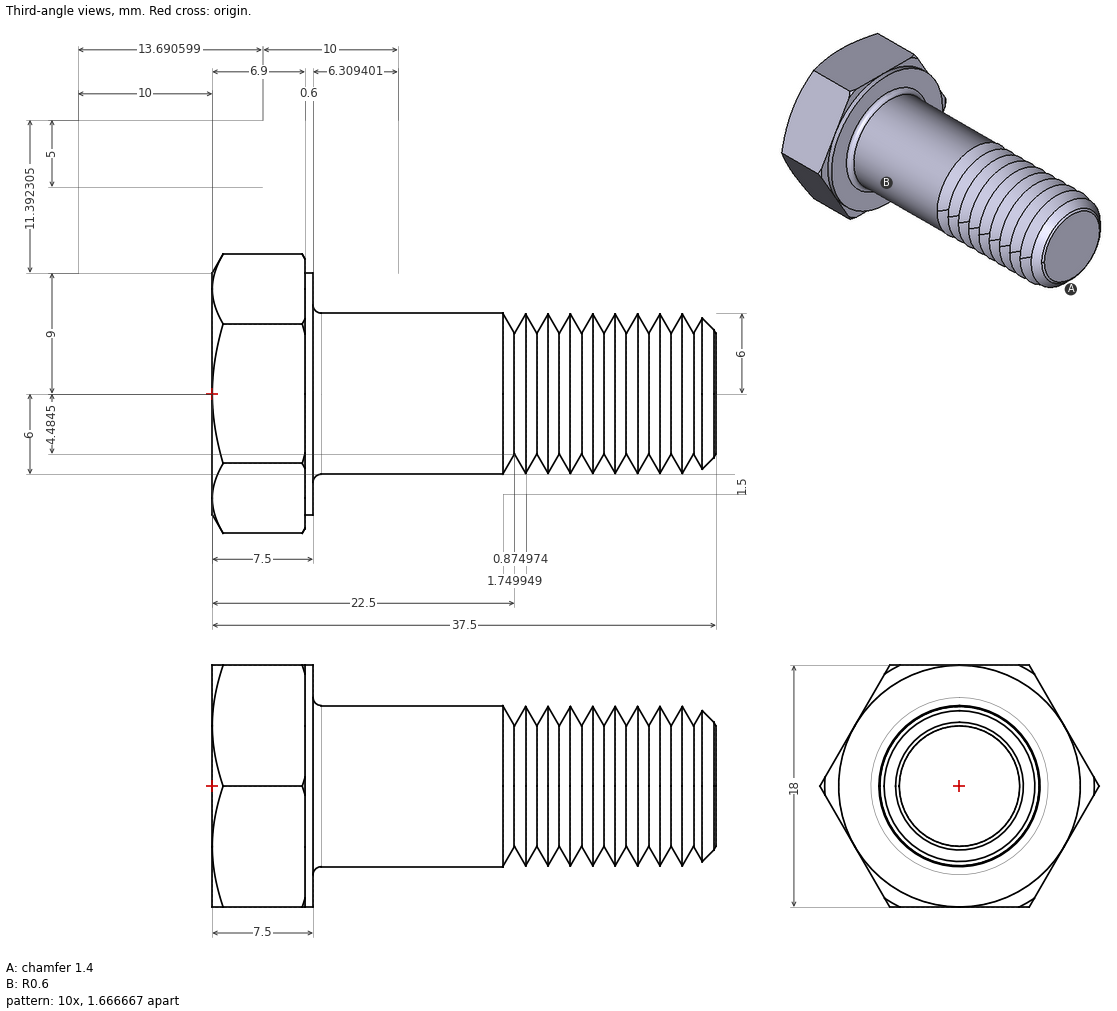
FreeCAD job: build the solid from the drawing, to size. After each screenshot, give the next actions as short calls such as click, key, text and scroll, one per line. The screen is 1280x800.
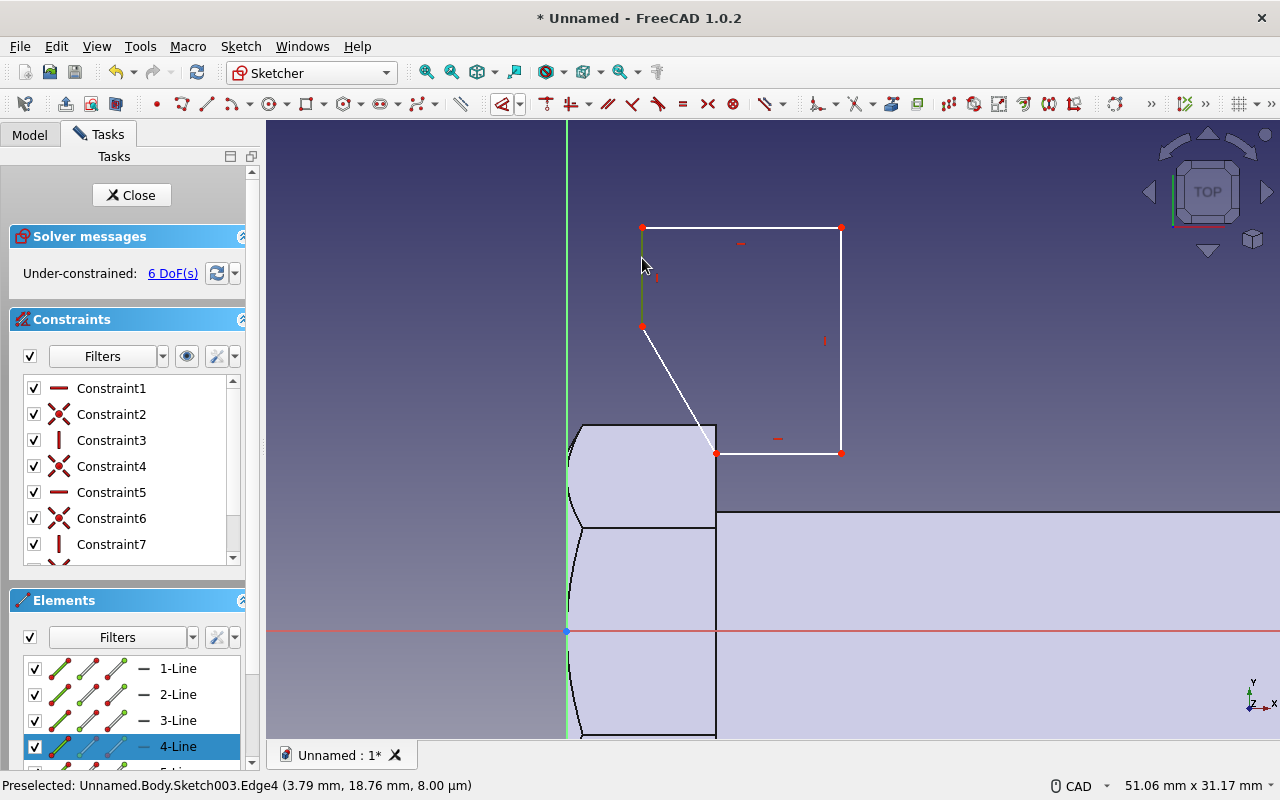
click(520, 104)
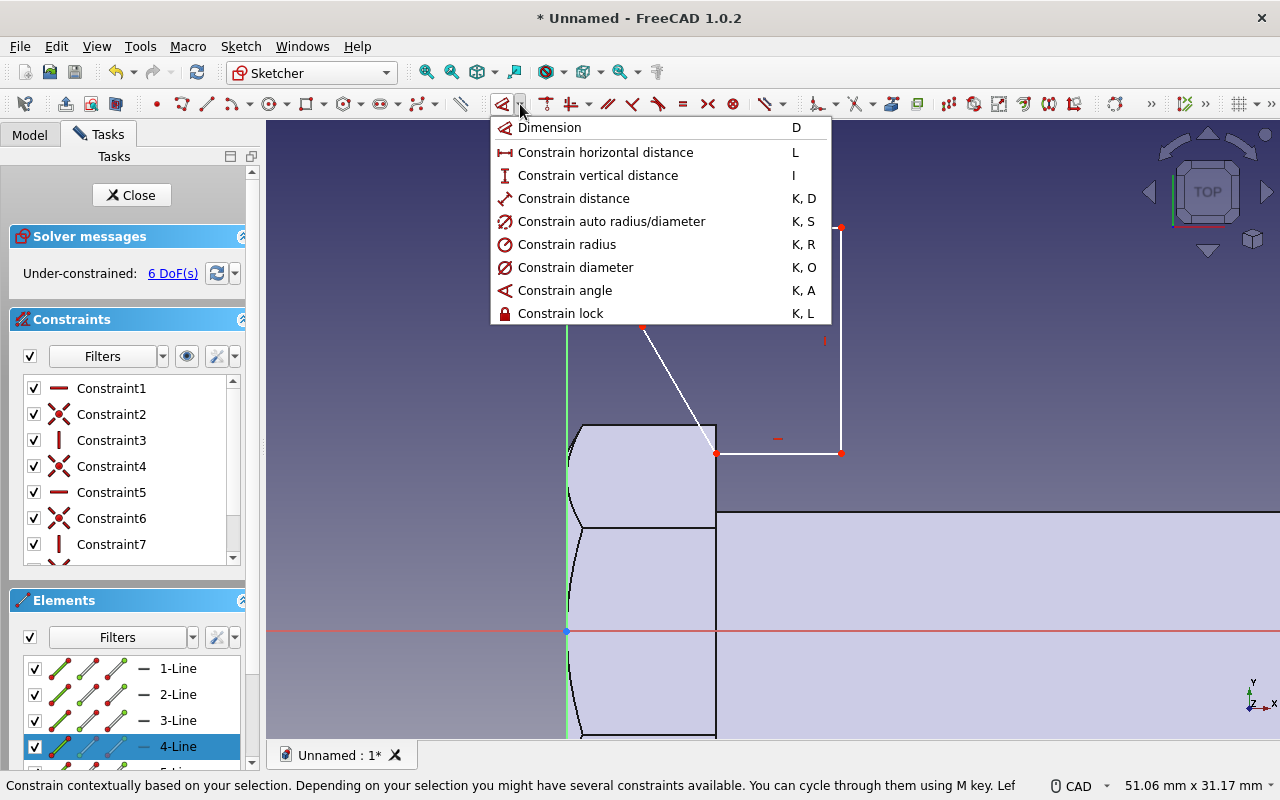
click(661, 176)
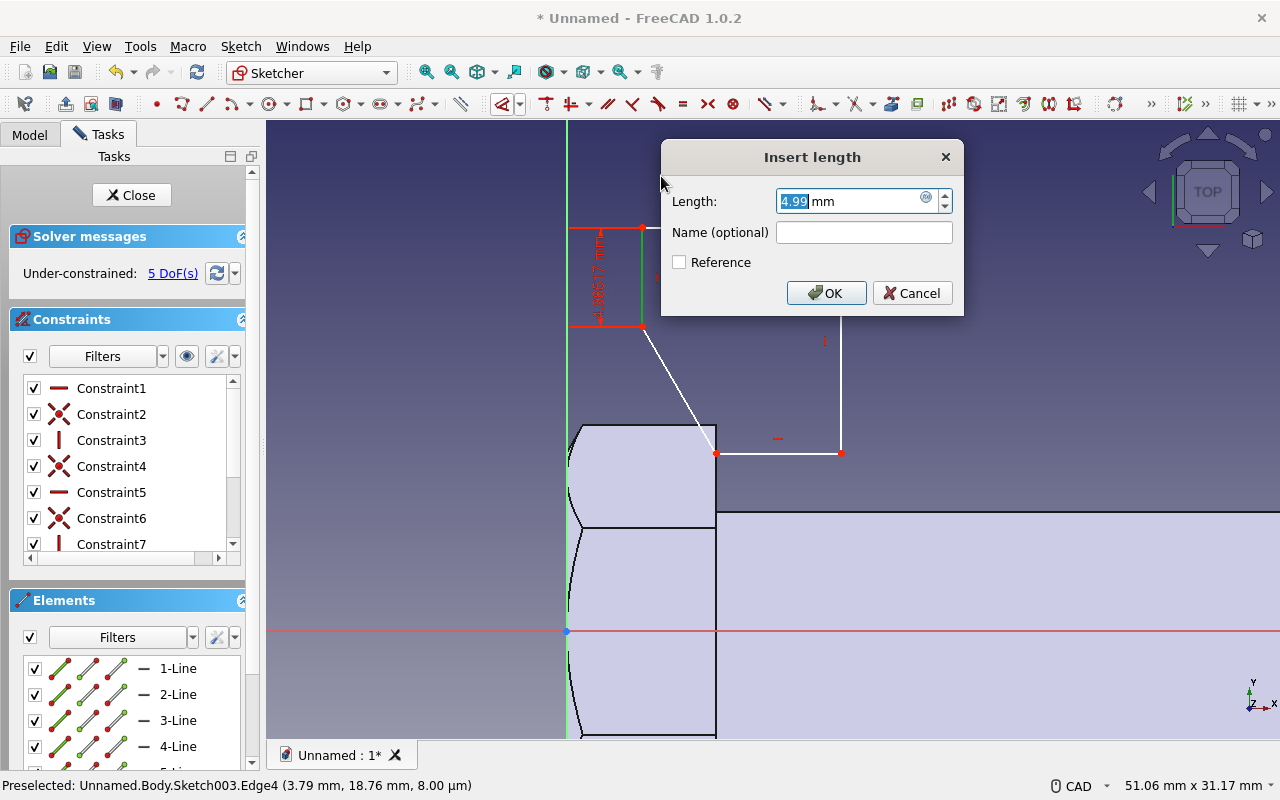
text(5)
key(Return)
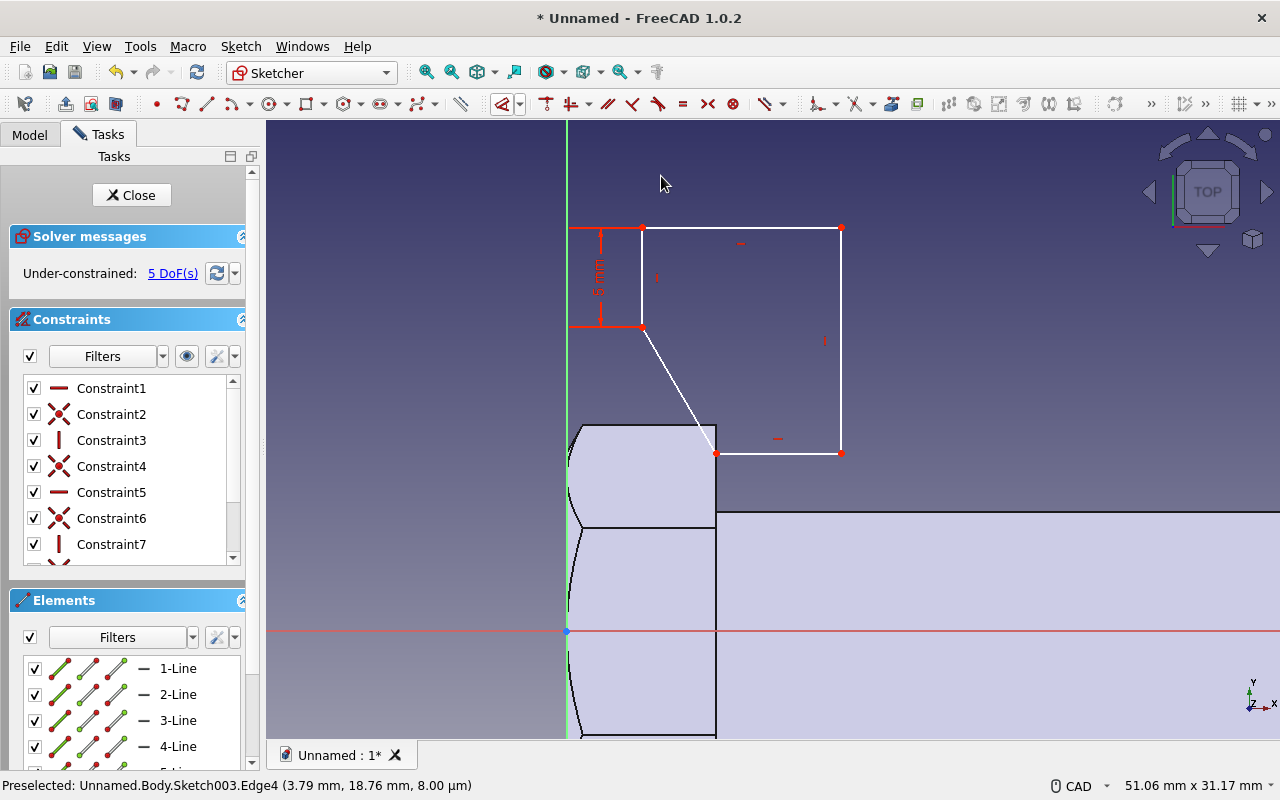
click(781, 228)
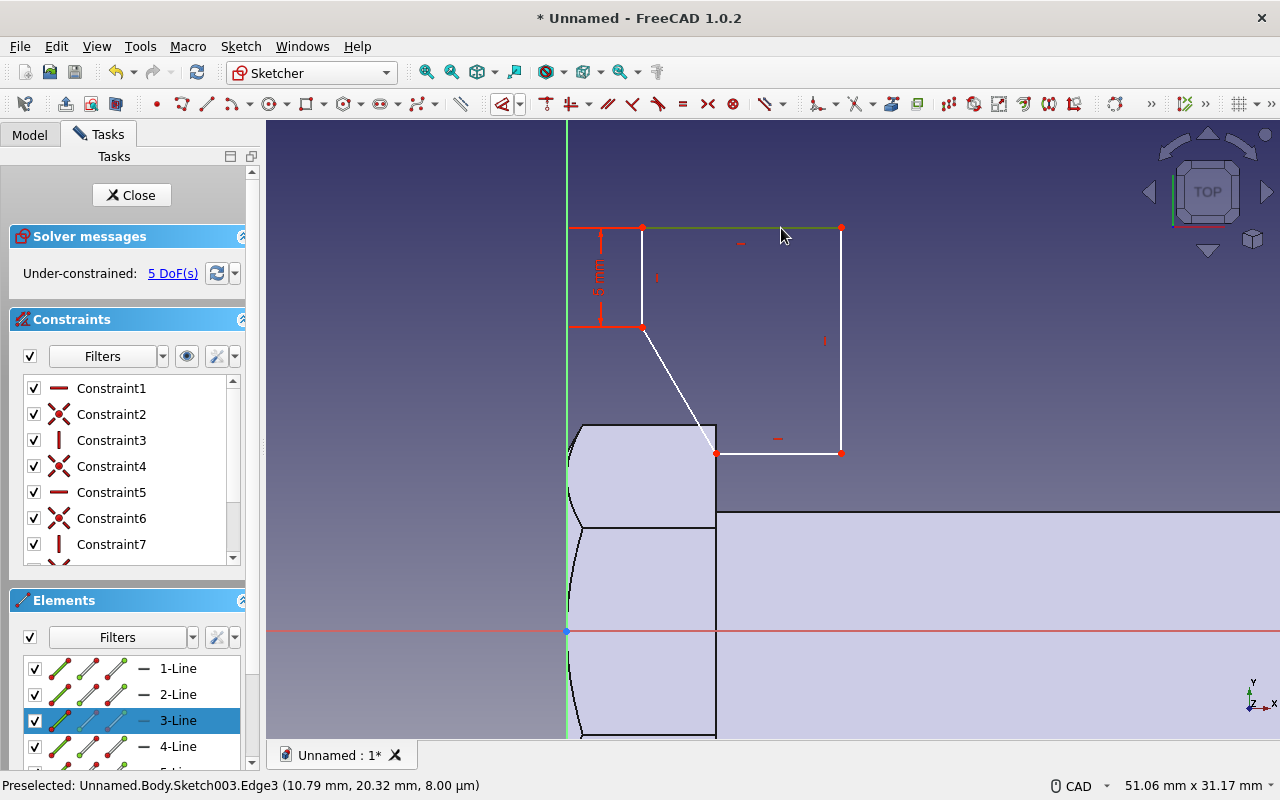
key(l)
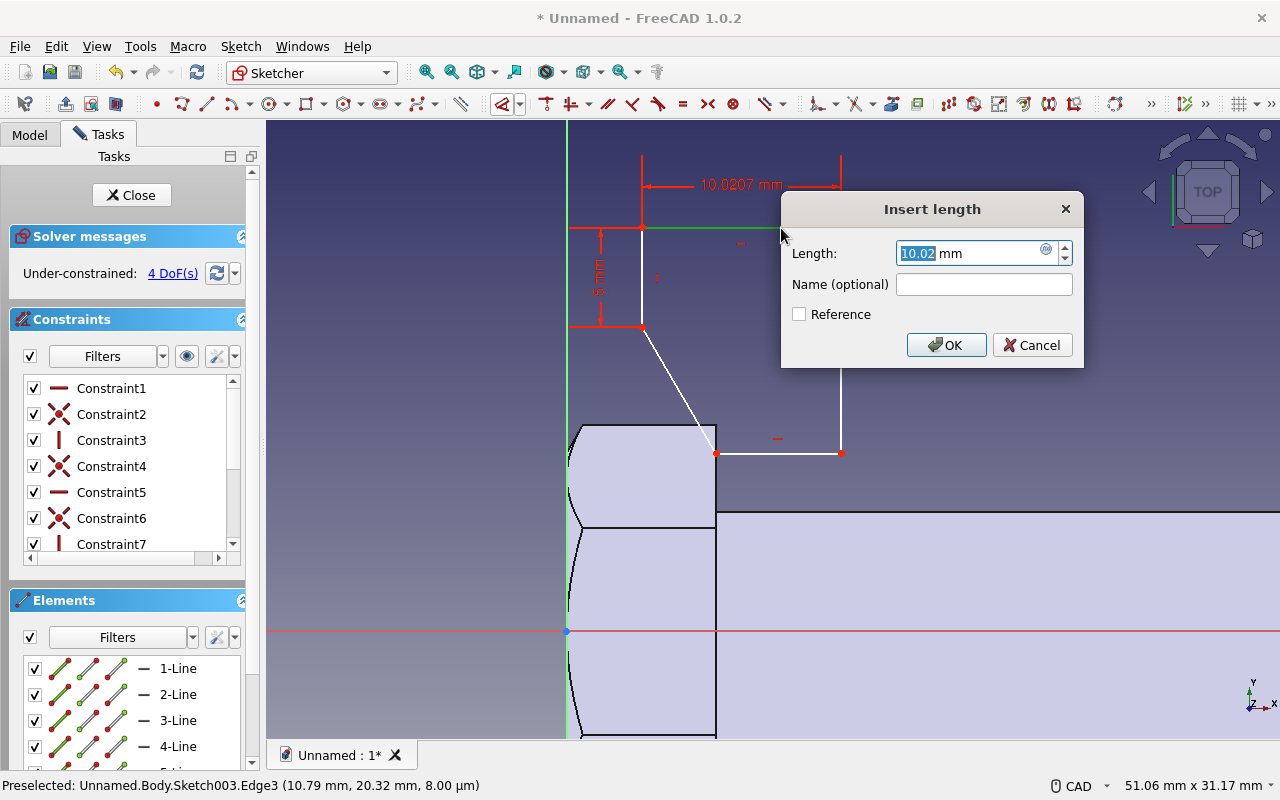
text(10)
key(Return)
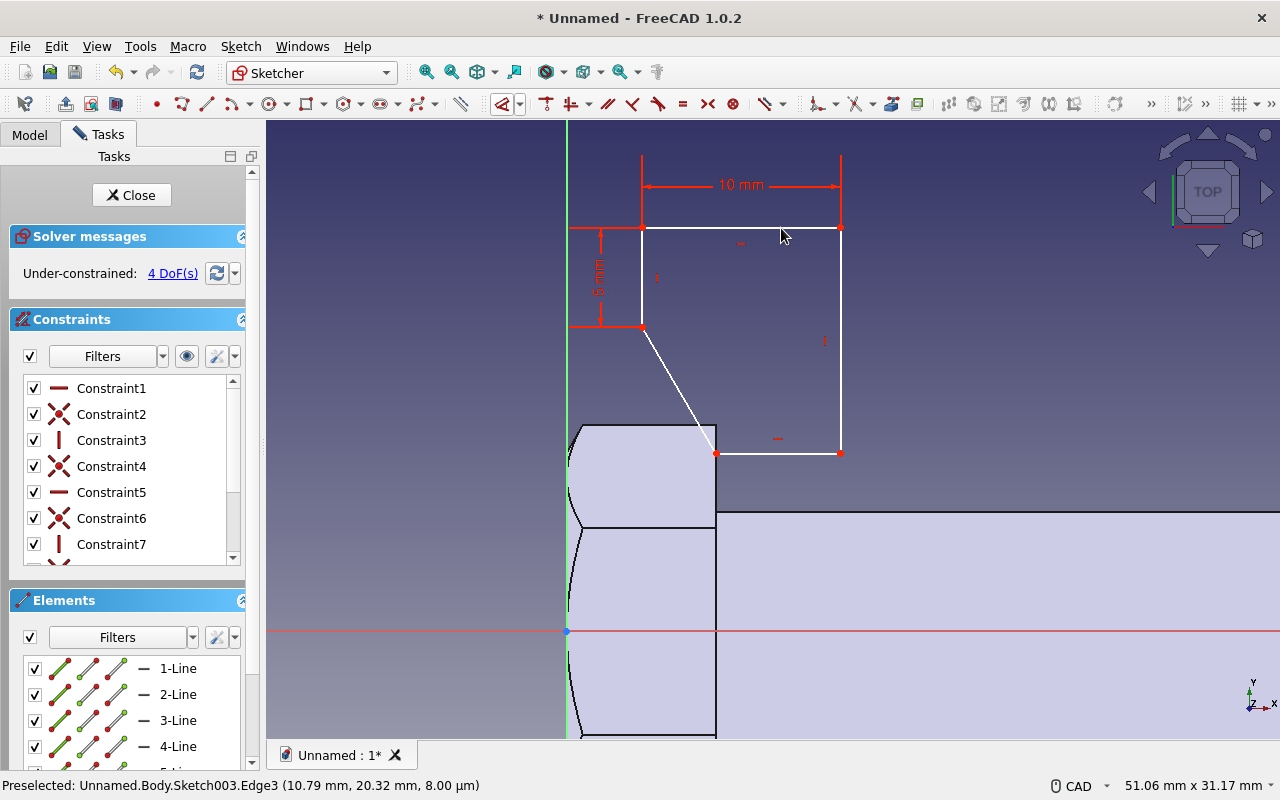
click(716, 454)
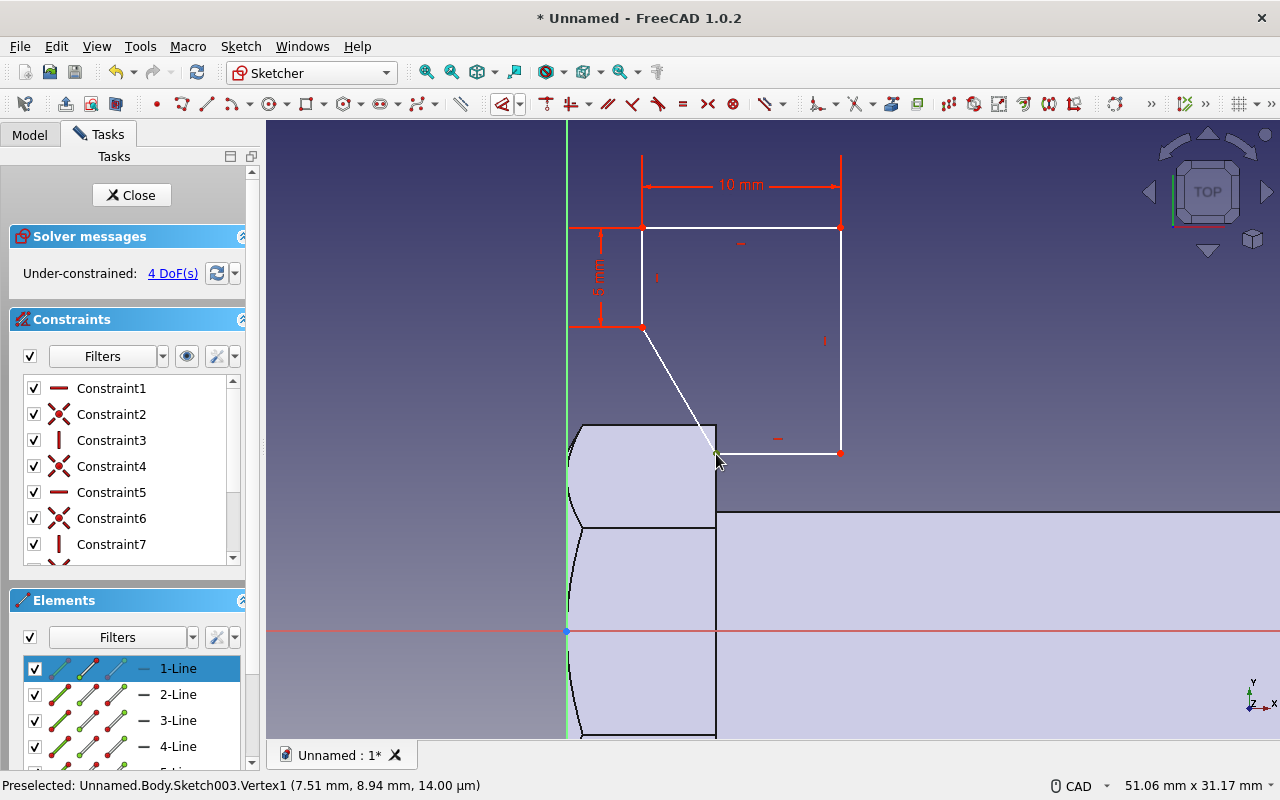
key(i)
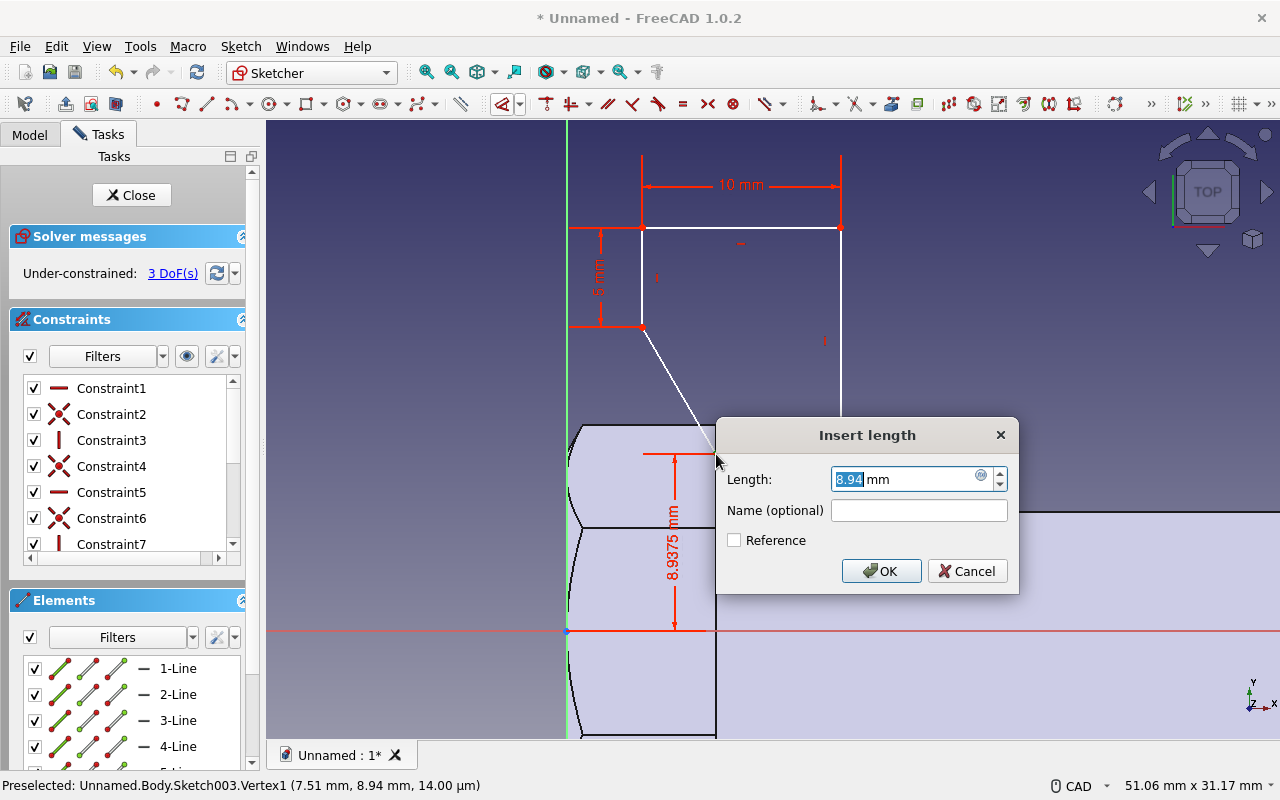
text(9)
key(Return)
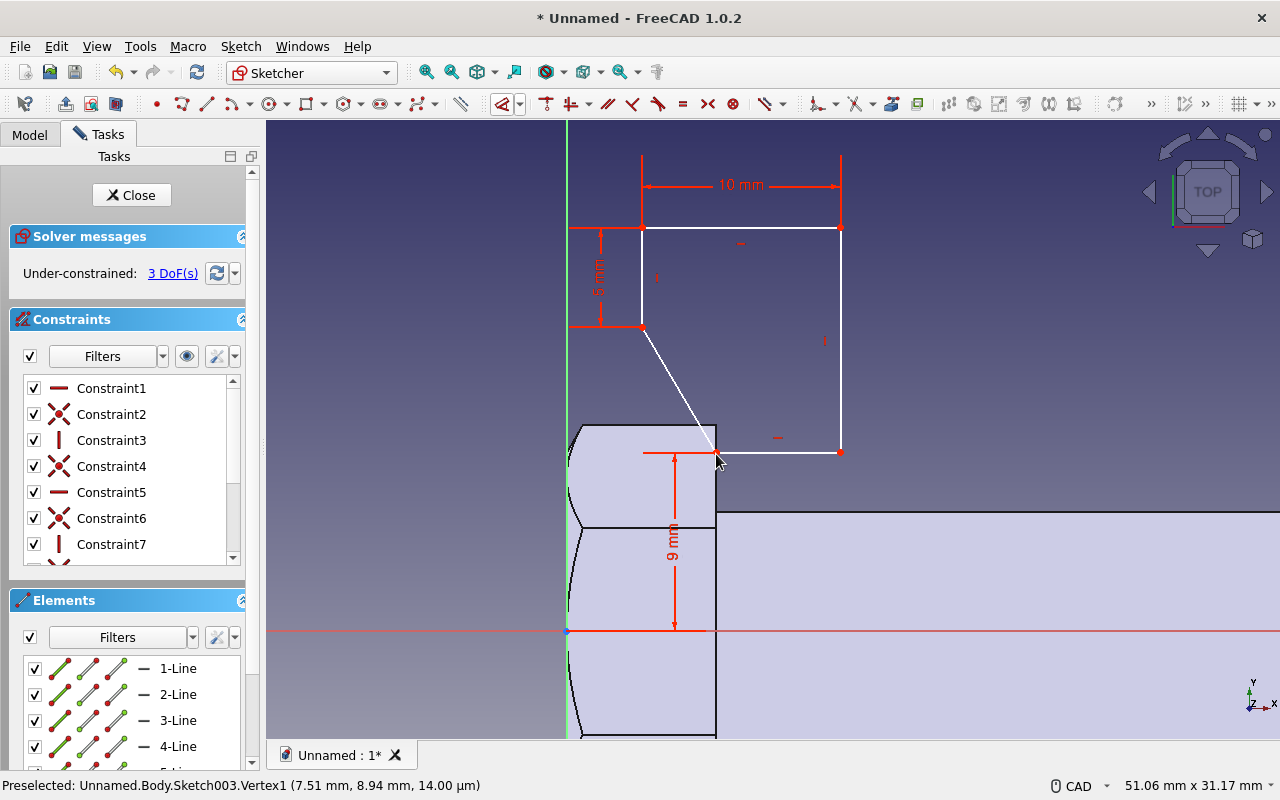
click(716, 453)